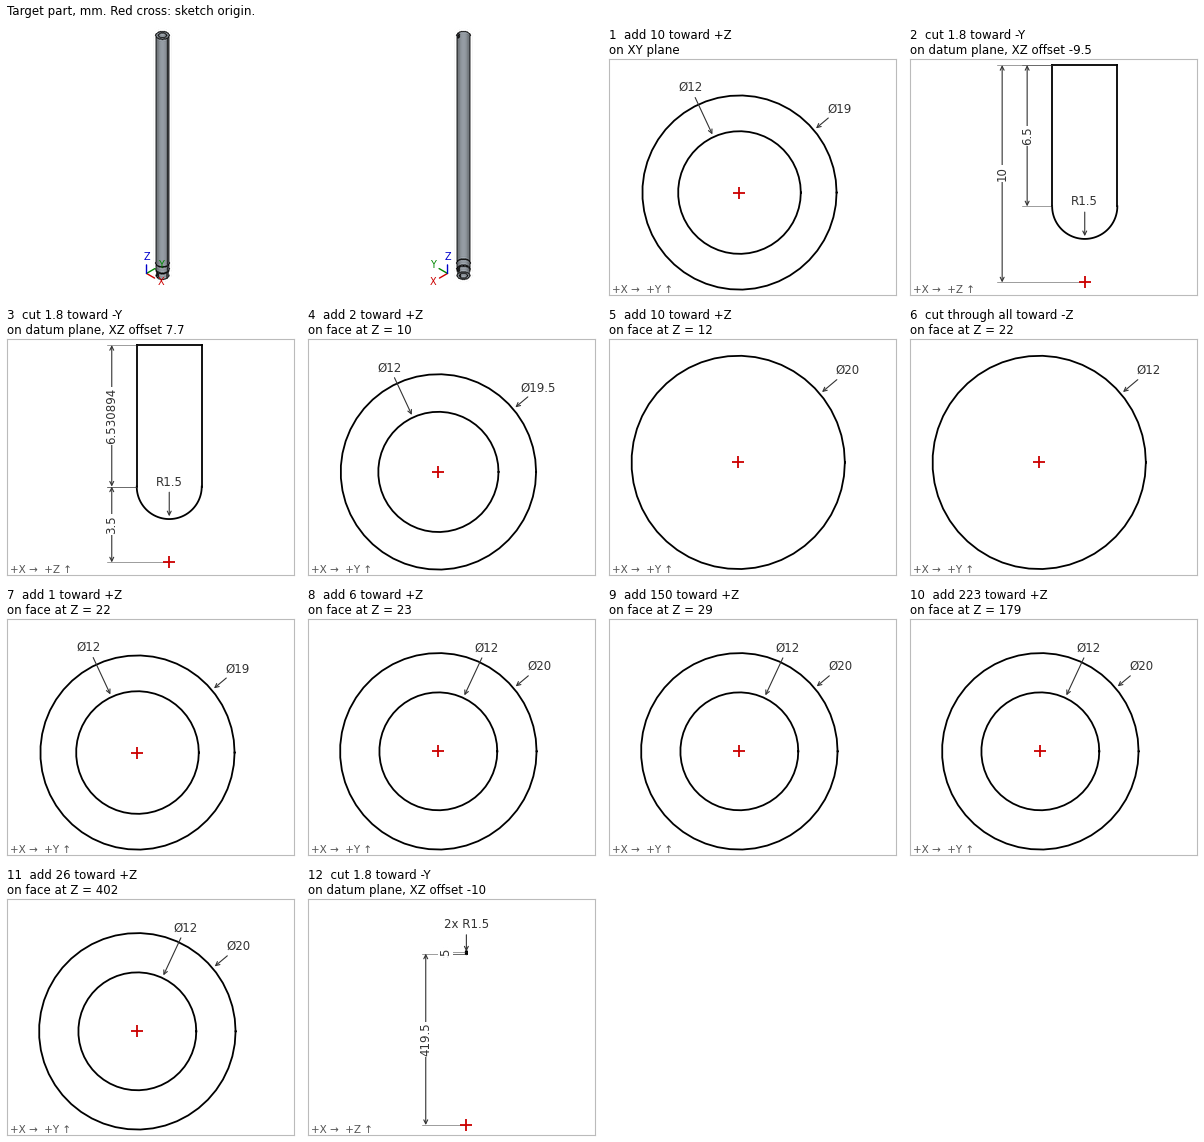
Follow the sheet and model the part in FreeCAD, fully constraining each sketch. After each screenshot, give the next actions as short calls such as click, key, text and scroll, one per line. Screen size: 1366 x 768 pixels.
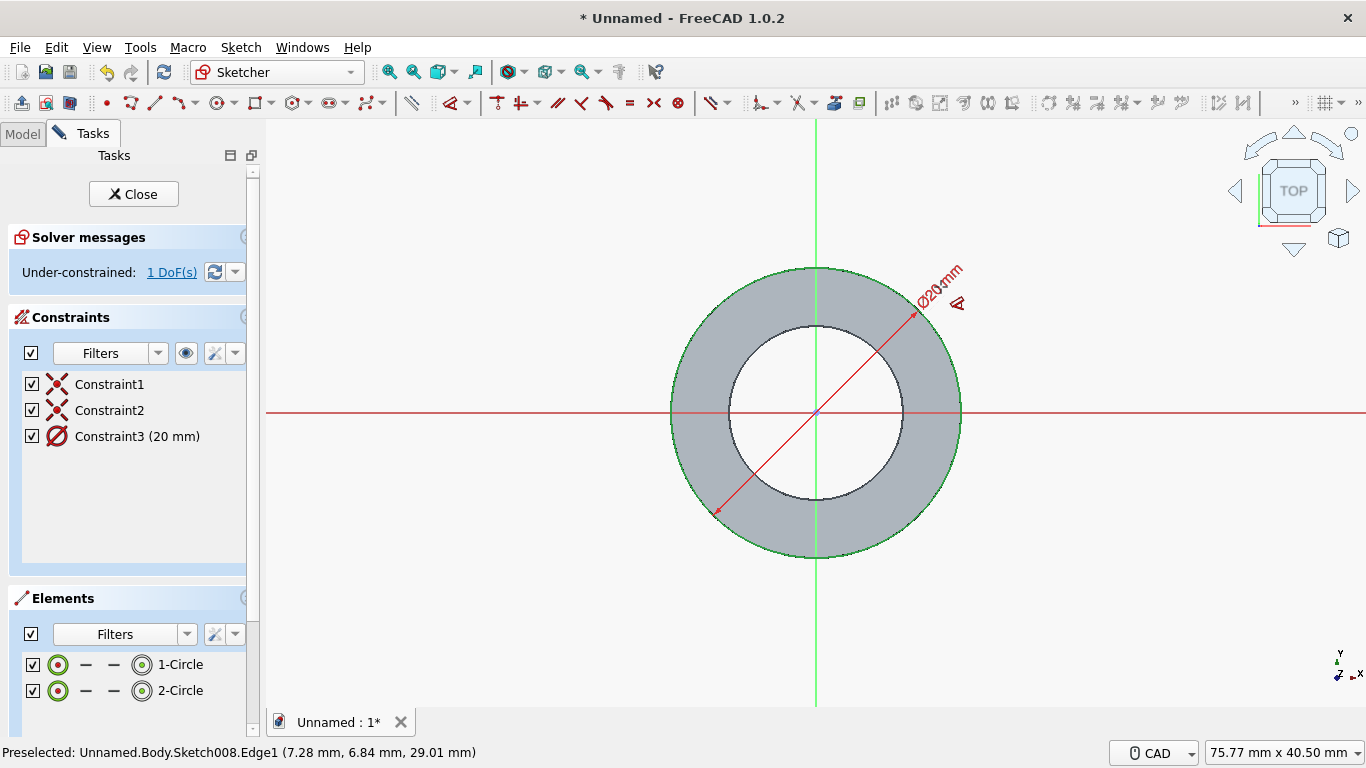
click(877, 351)
click(899, 328)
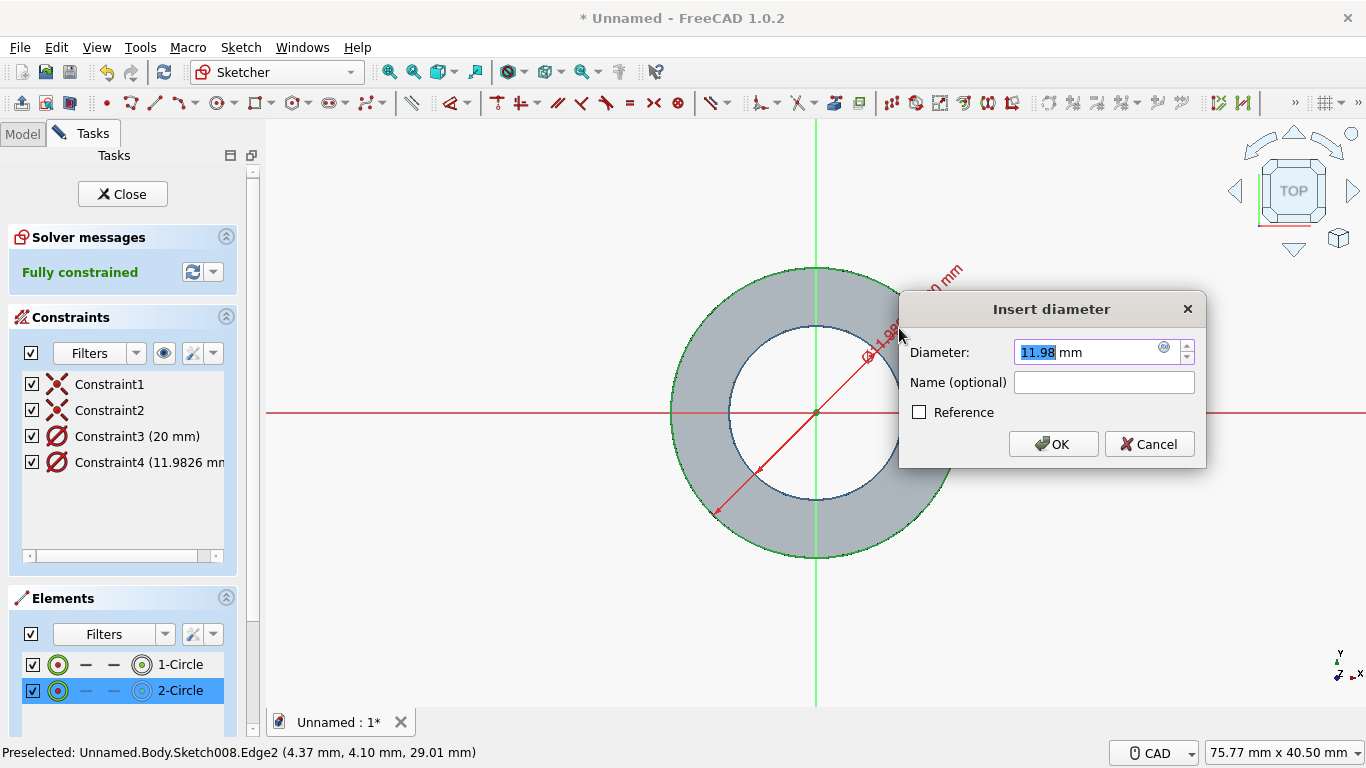
text(12)
key(Return)
key(Escape)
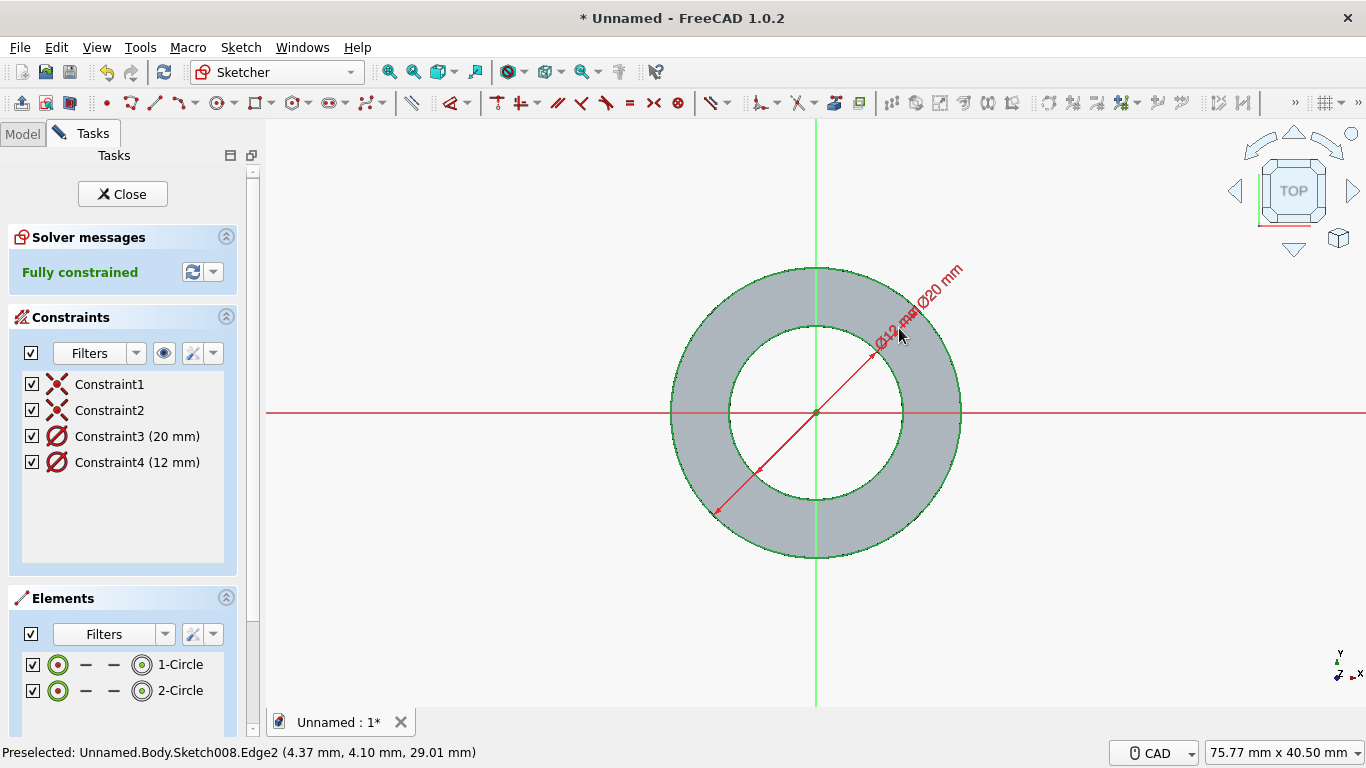
click(123, 194)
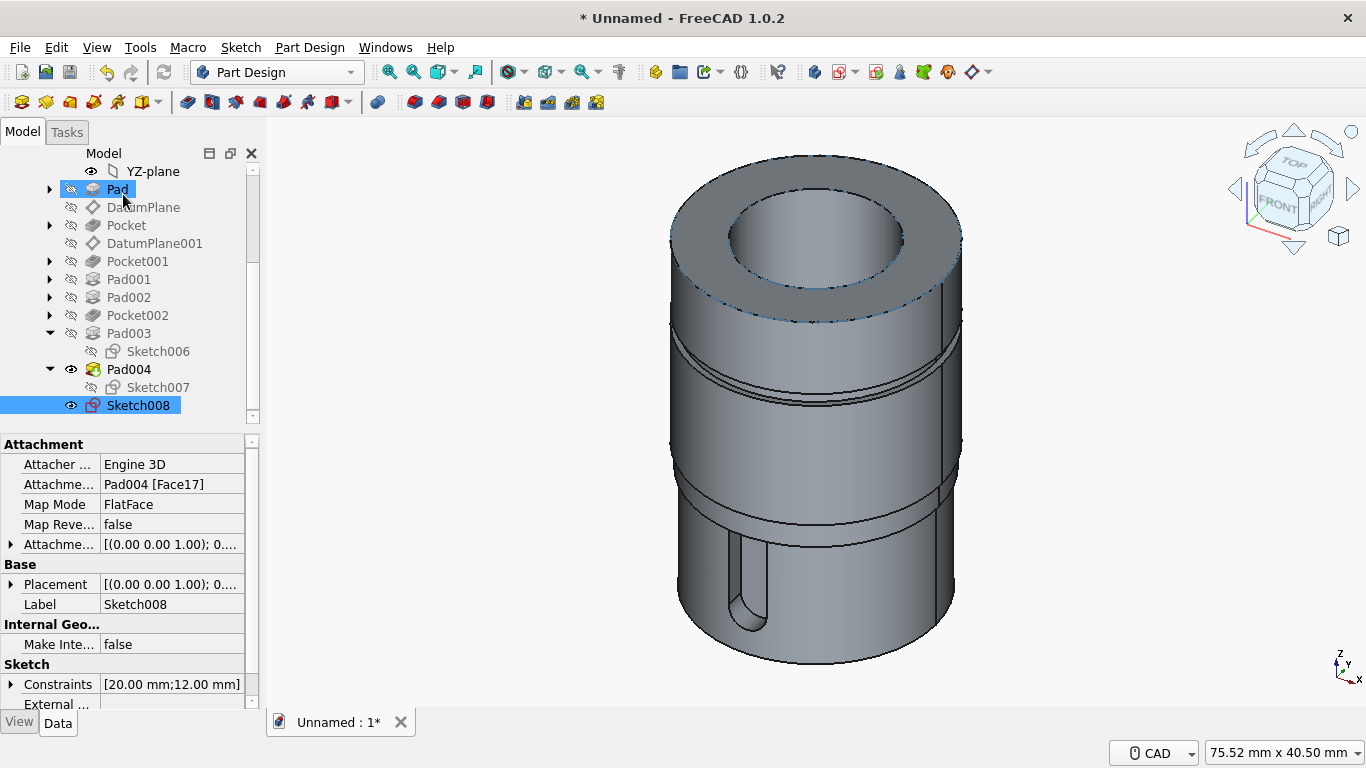
click(22, 102)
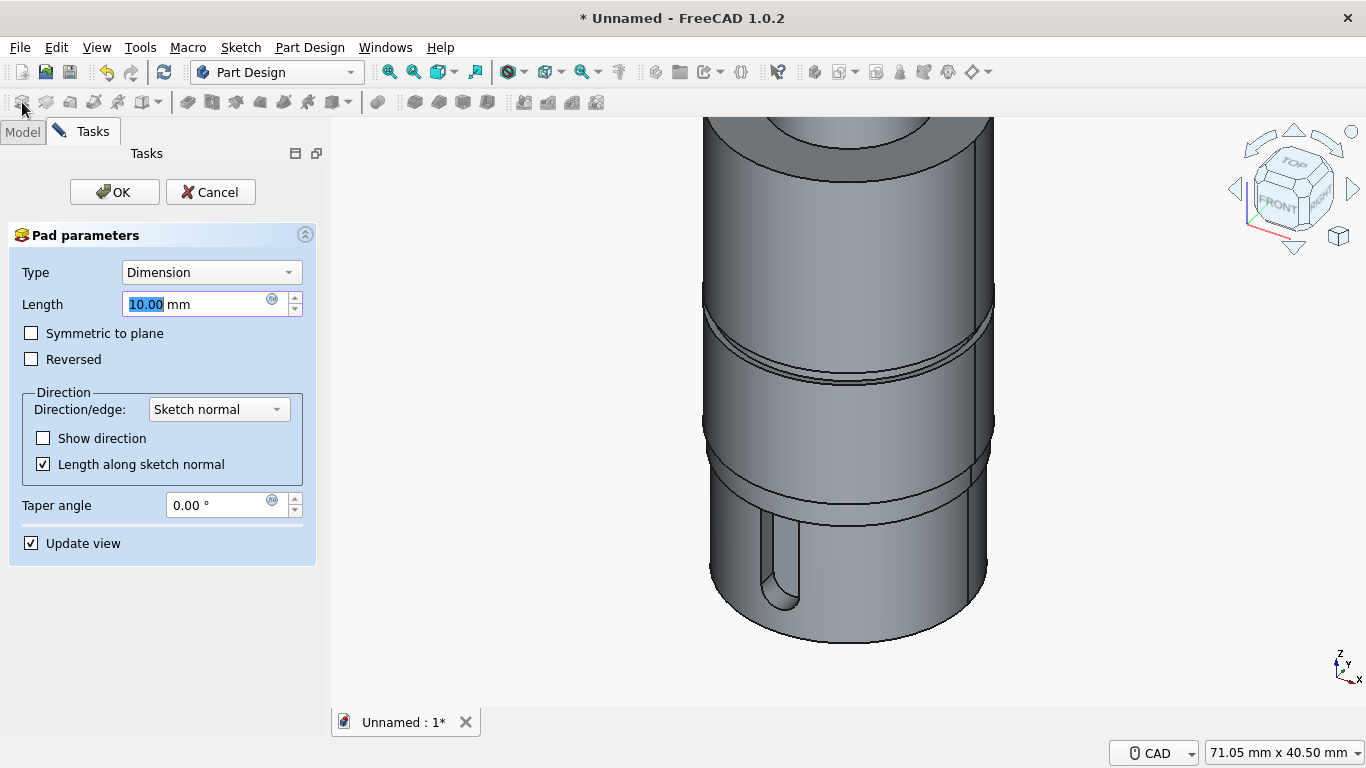
text(150)
key(Tab)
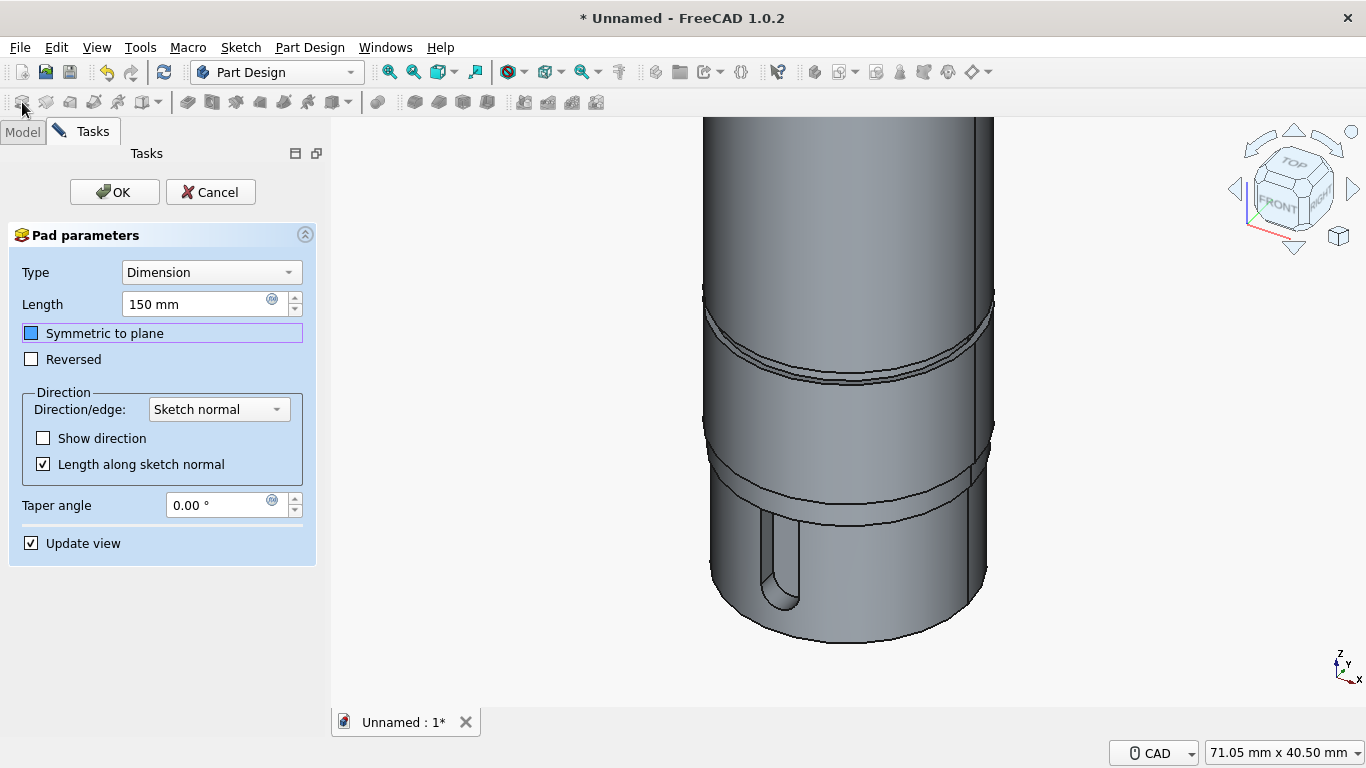
click(115, 192)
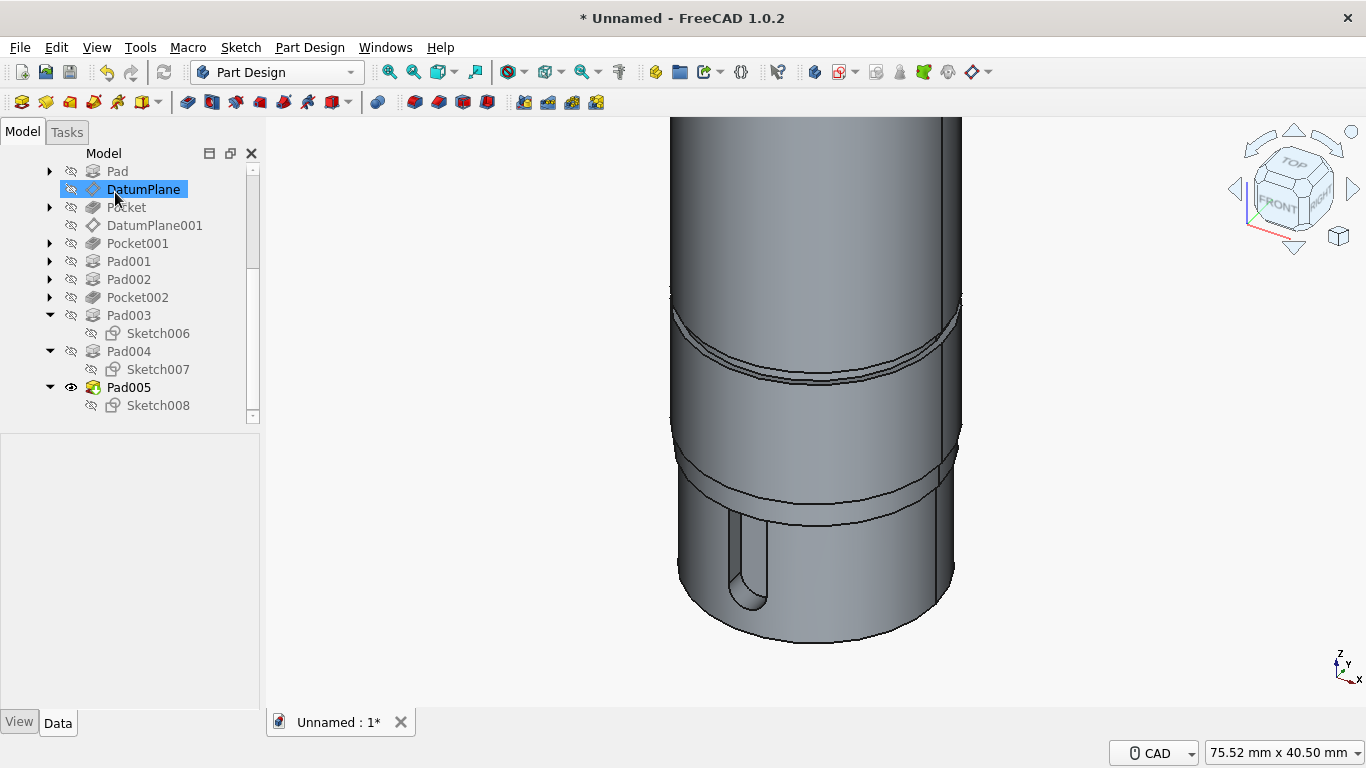
click(390, 72)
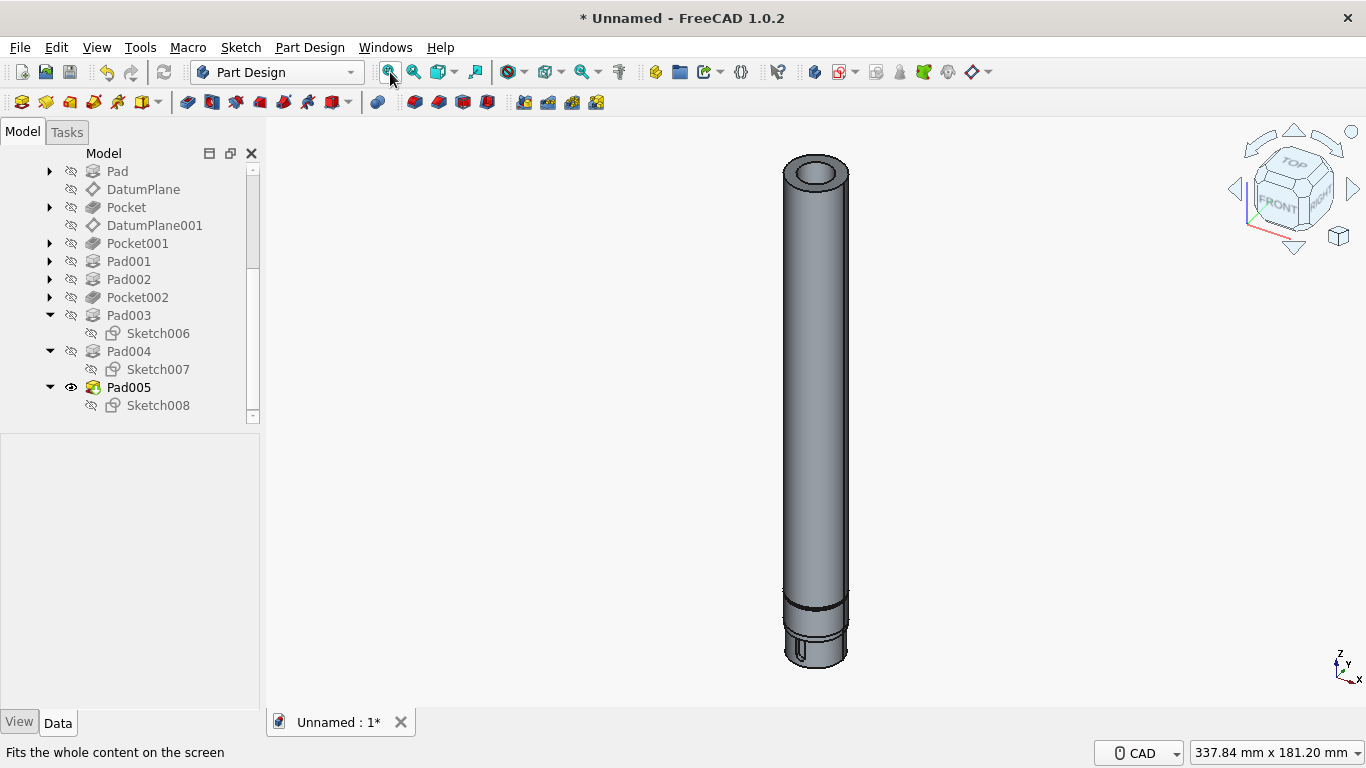
scroll(841, 168, up, 4)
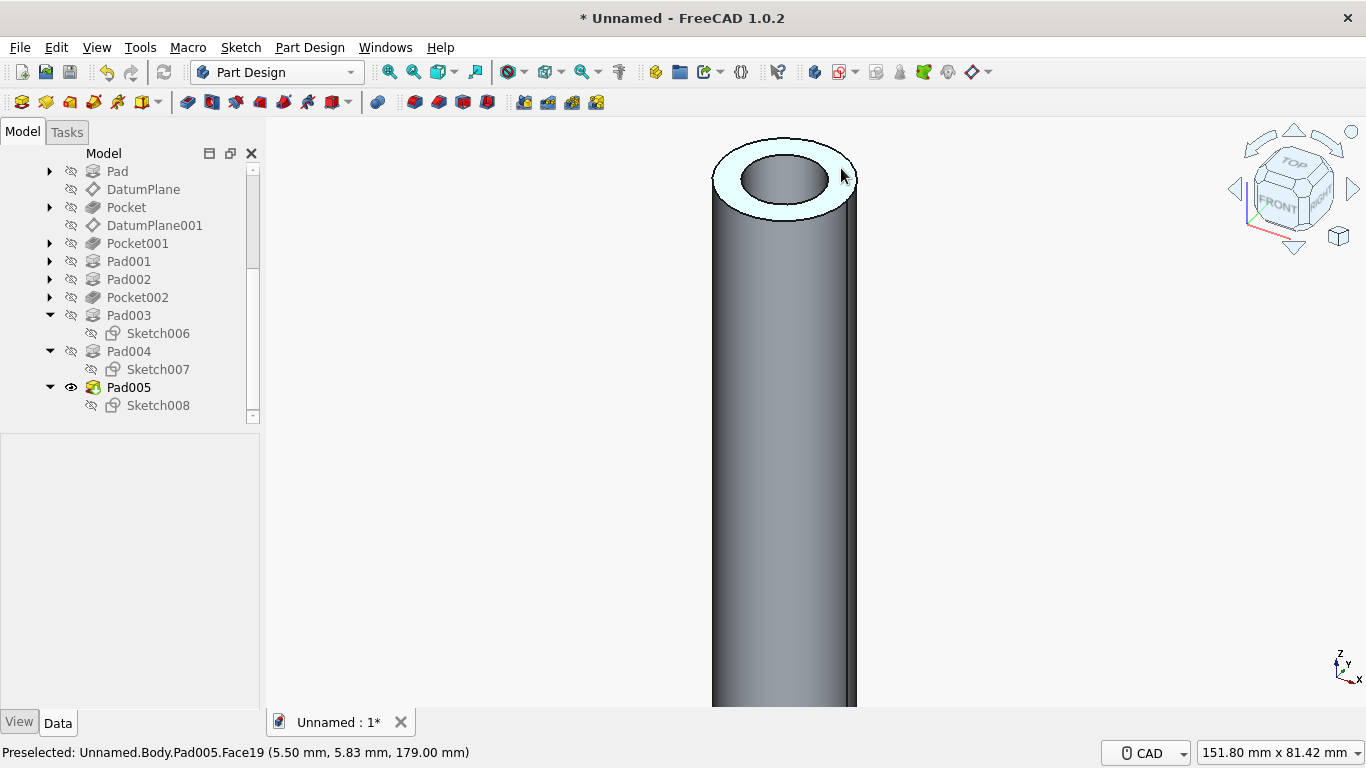
click(841, 170)